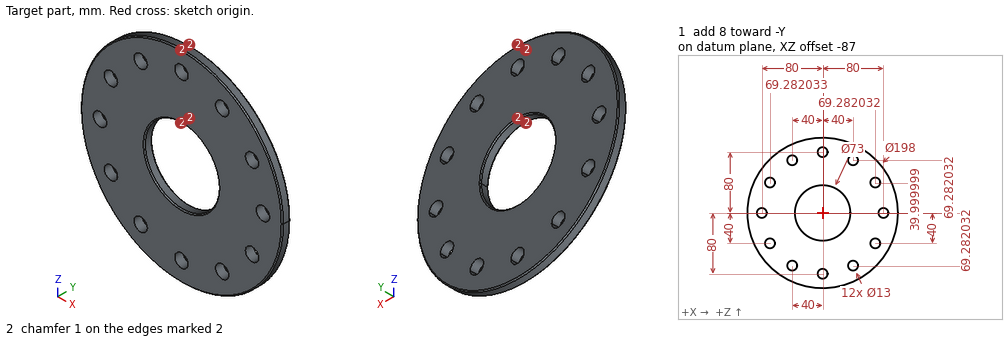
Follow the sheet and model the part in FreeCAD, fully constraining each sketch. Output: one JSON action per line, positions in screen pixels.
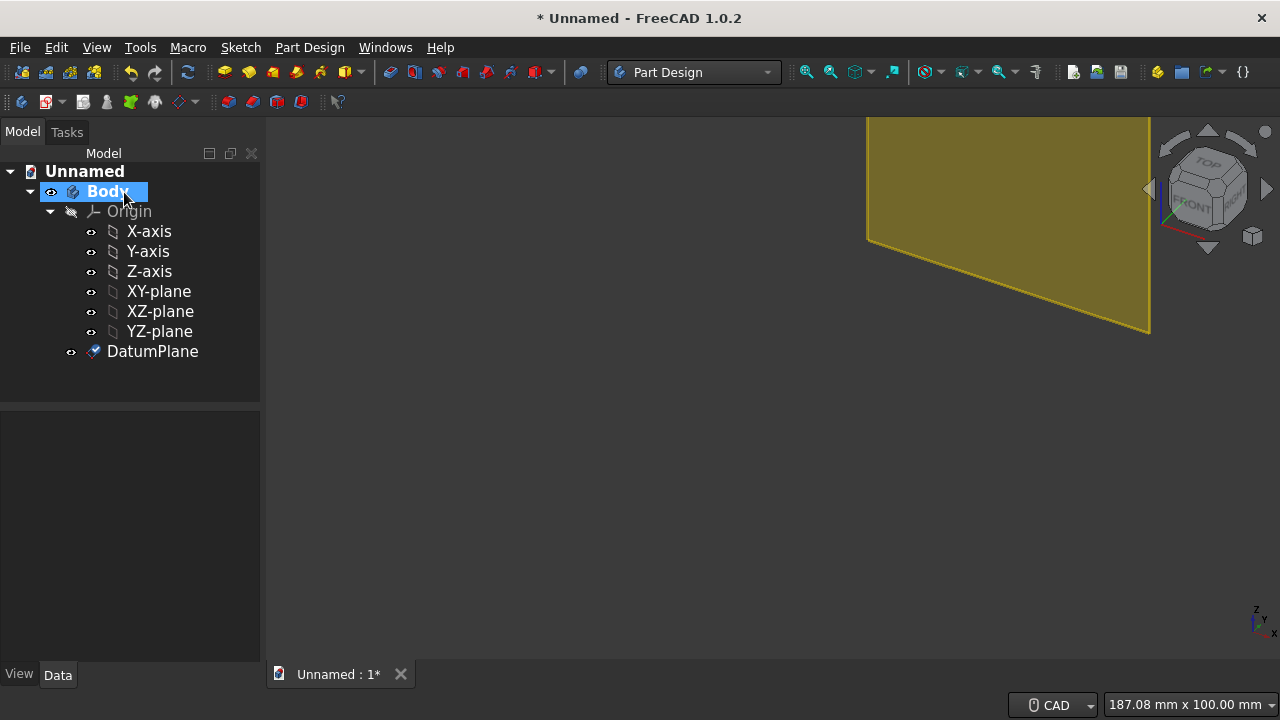
{"action": "left_click", "coordinate": [116, 352]}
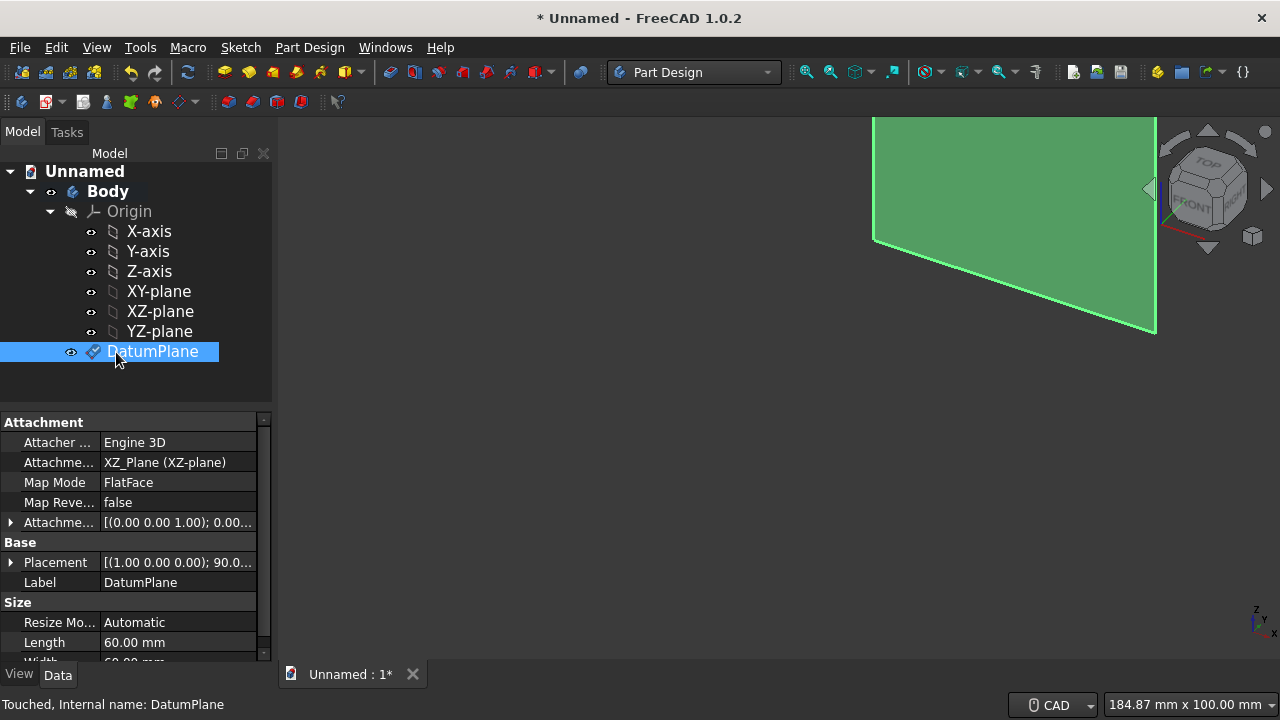
{"action": "left_click", "coordinate": [46, 102]}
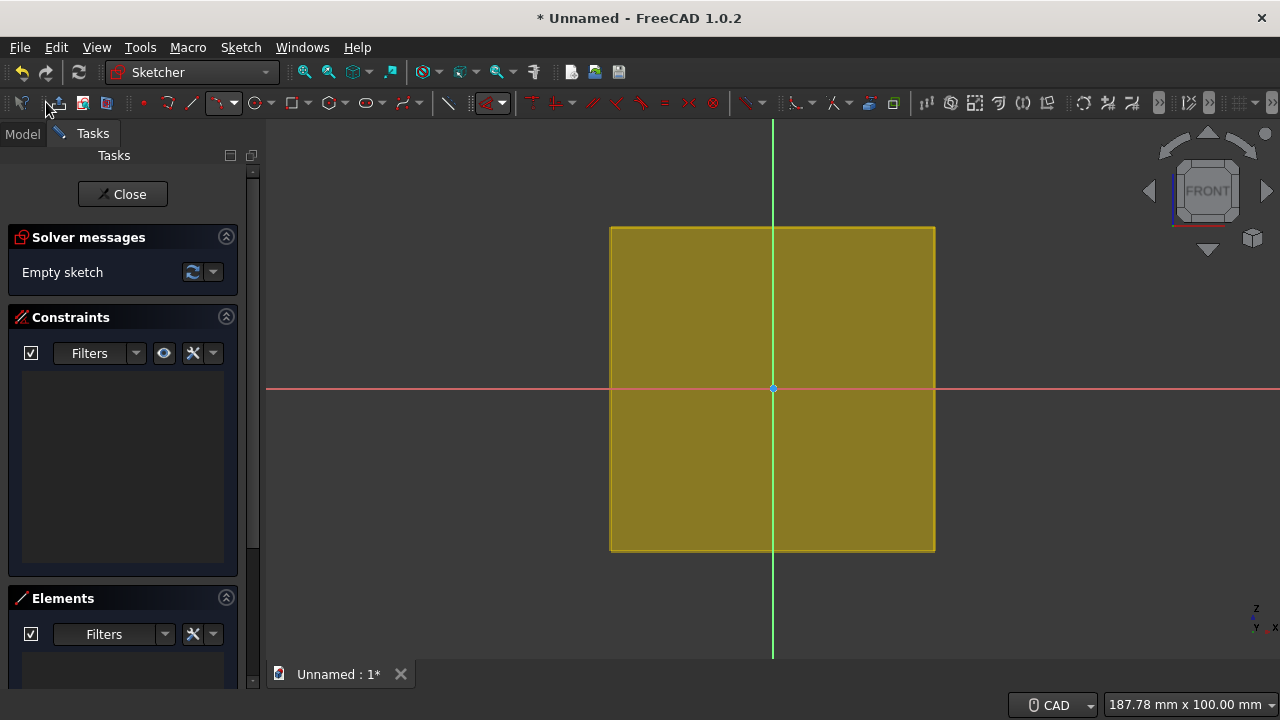
{"action": "scroll", "coordinate": [675, 389], "scroll_direction": "down", "scroll_amount": 6}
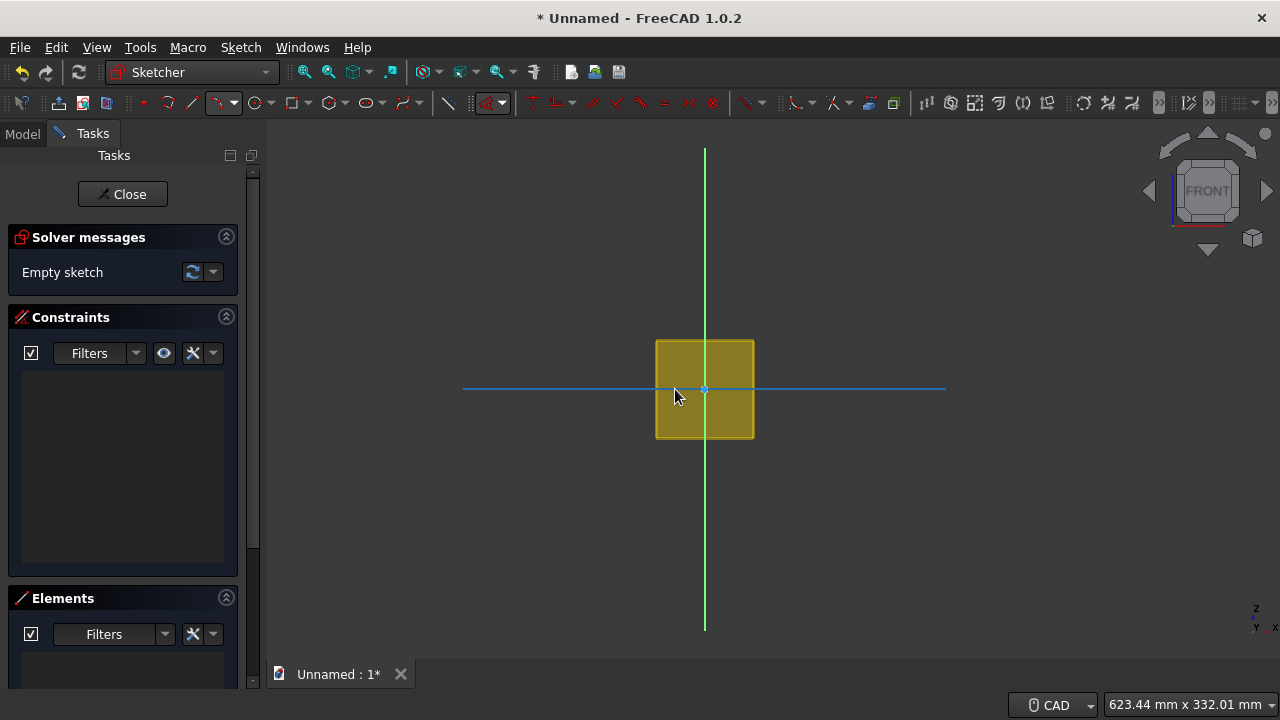
{"action": "key", "text": "g c"}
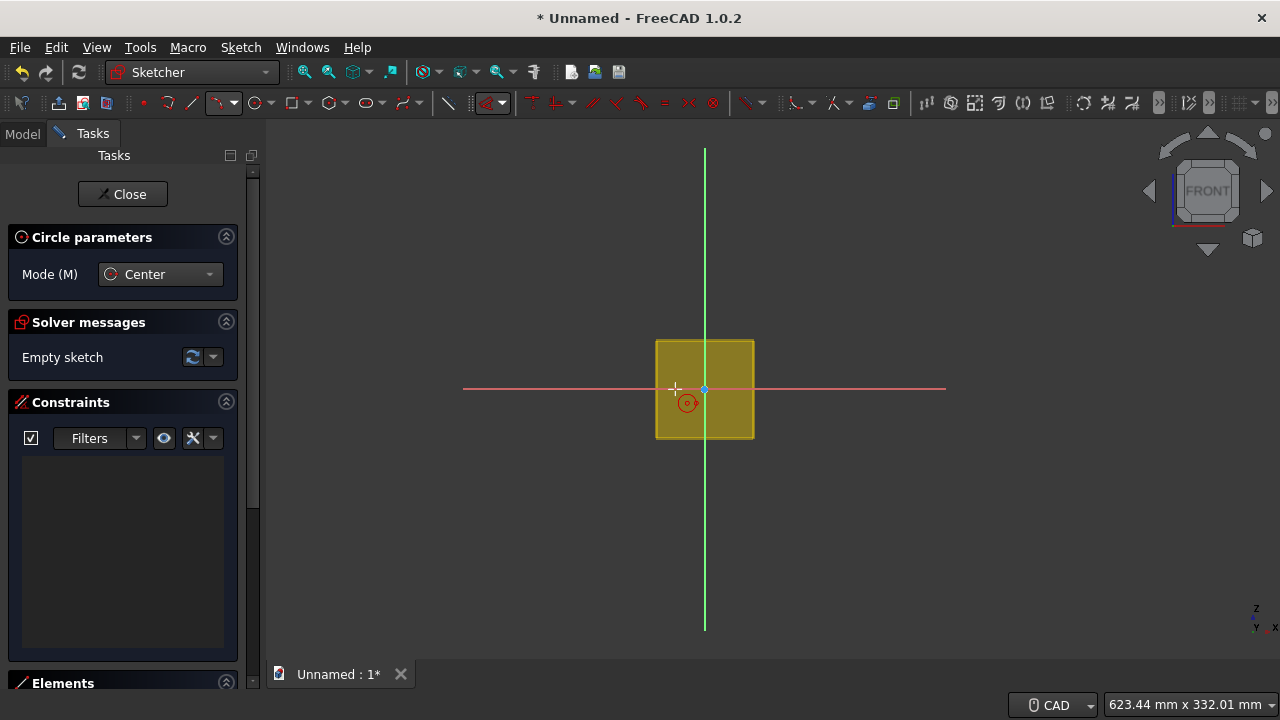
{"action": "left_click", "coordinate": [705, 389]}
{"action": "left_click", "coordinate": [819, 275]}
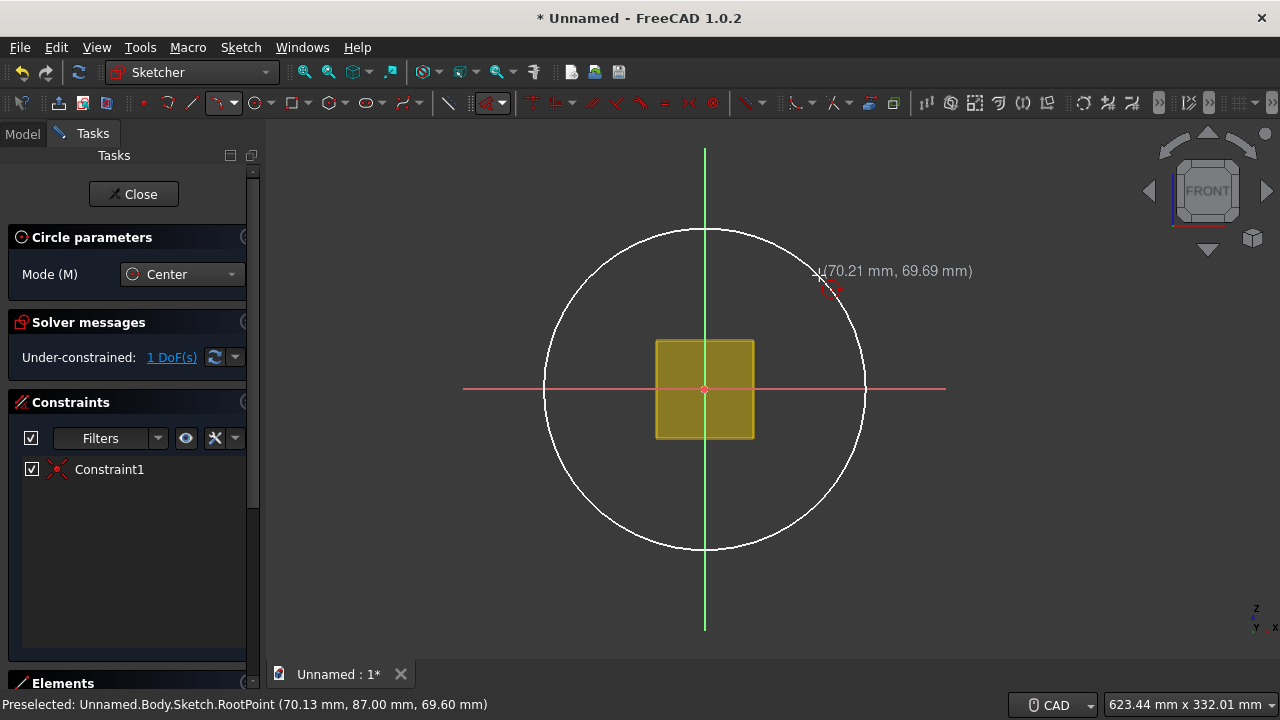
{"action": "scroll", "coordinate": [817, 324], "scroll_direction": "up", "scroll_amount": 4}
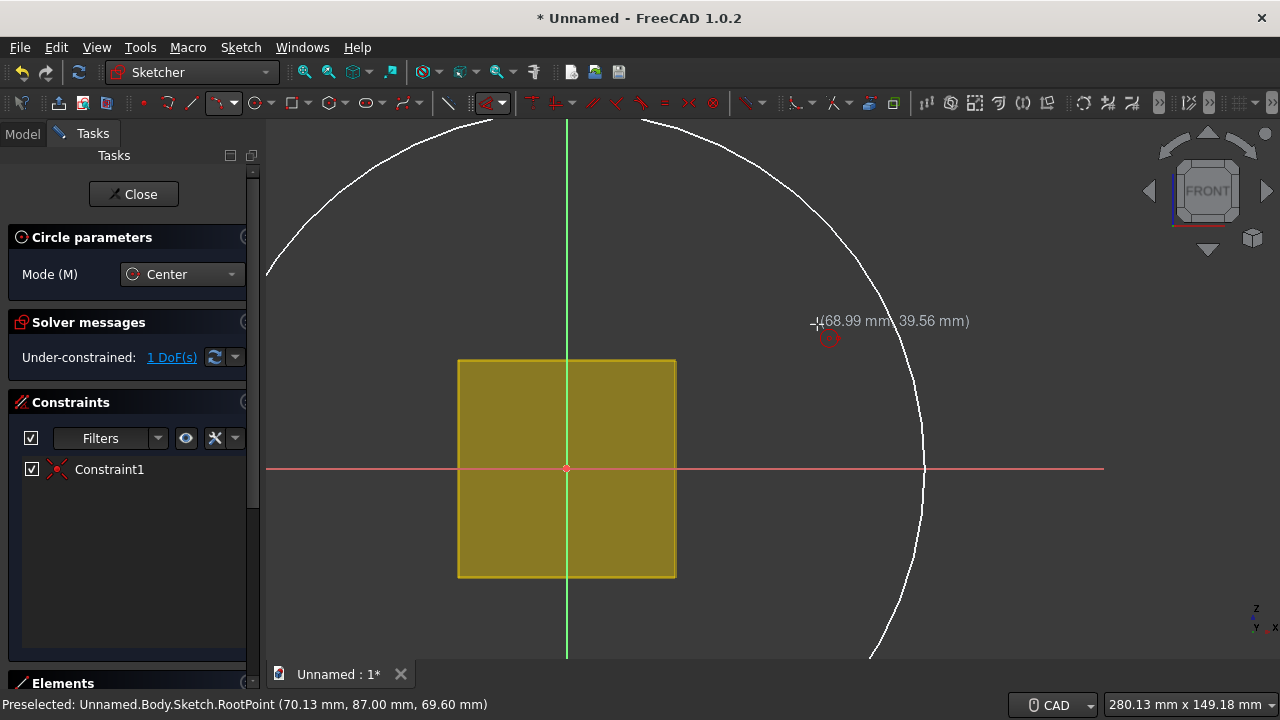
{"action": "left_click", "coordinate": [817, 324]}
{"action": "left_click", "coordinate": [834, 308]}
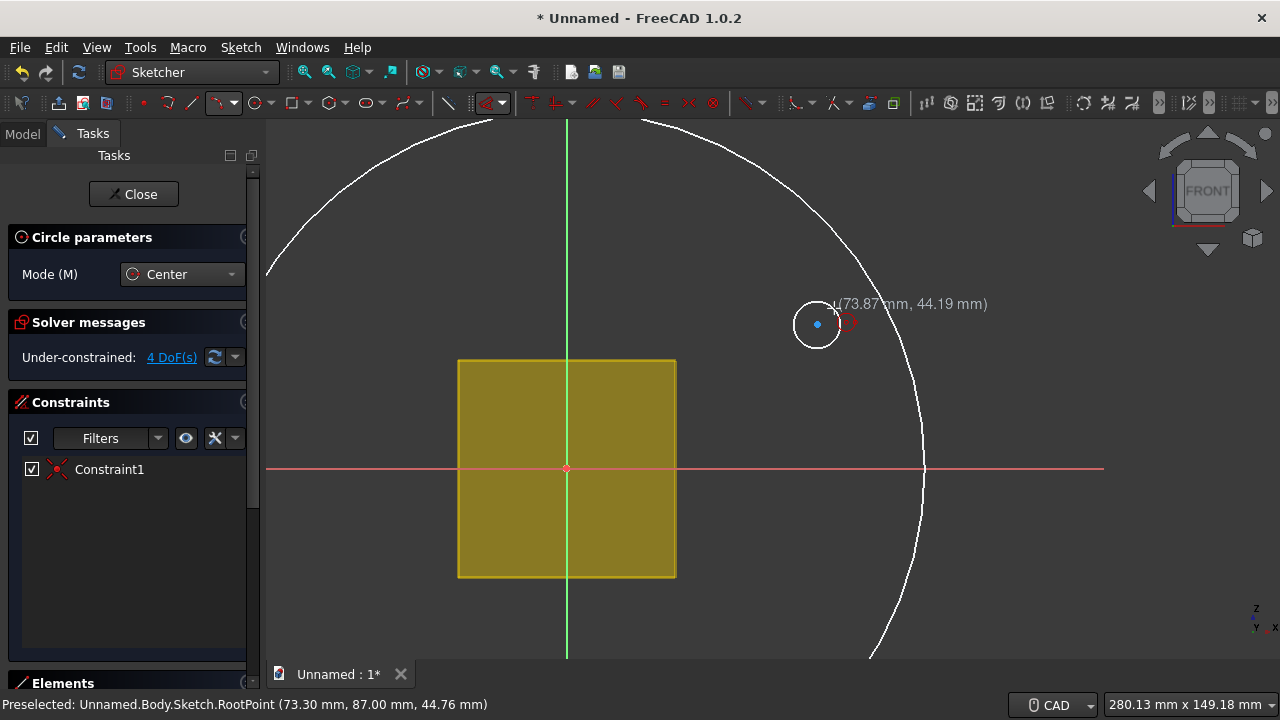
{"action": "left_click", "coordinate": [711, 218]}
{"action": "left_click", "coordinate": [728, 202]}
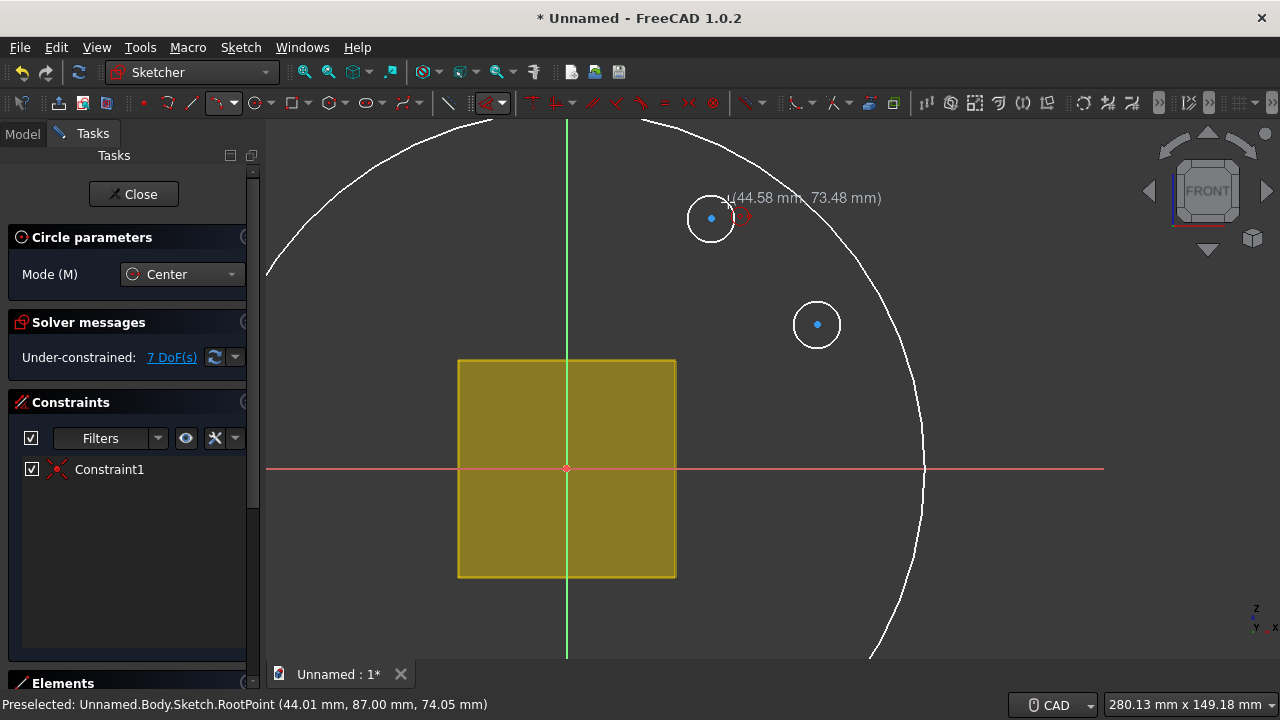
{"action": "left_click", "coordinate": [567, 179]}
{"action": "left_click", "coordinate": [583, 163]}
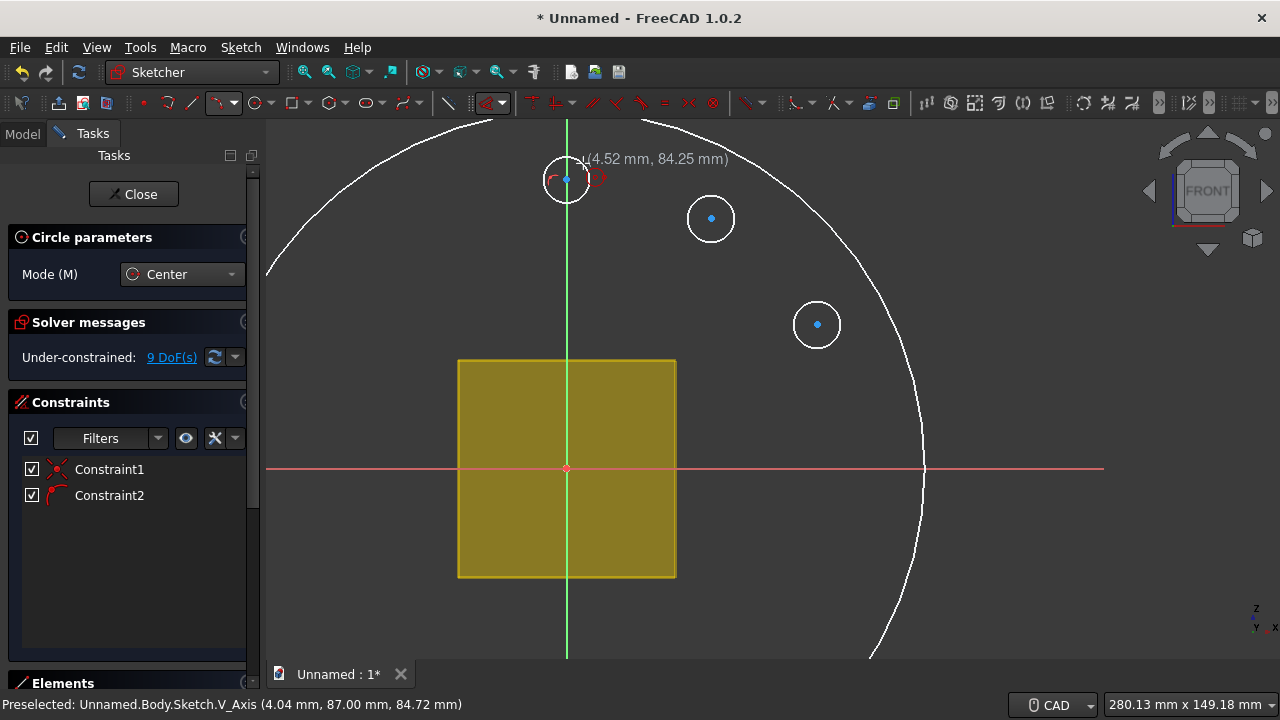
{"action": "left_click", "coordinate": [856, 469]}
{"action": "left_click", "coordinate": [873, 452]}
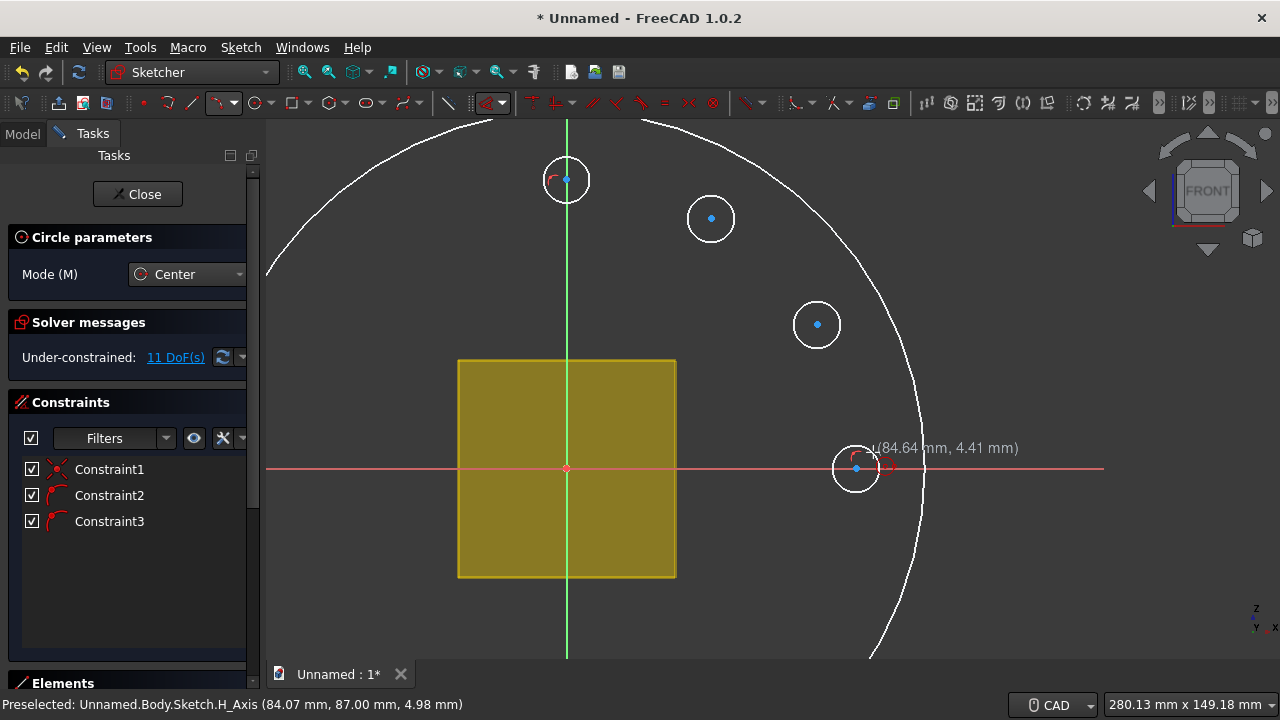
{"action": "left_click", "coordinate": [817, 614]}
{"action": "left_click", "coordinate": [834, 597]}